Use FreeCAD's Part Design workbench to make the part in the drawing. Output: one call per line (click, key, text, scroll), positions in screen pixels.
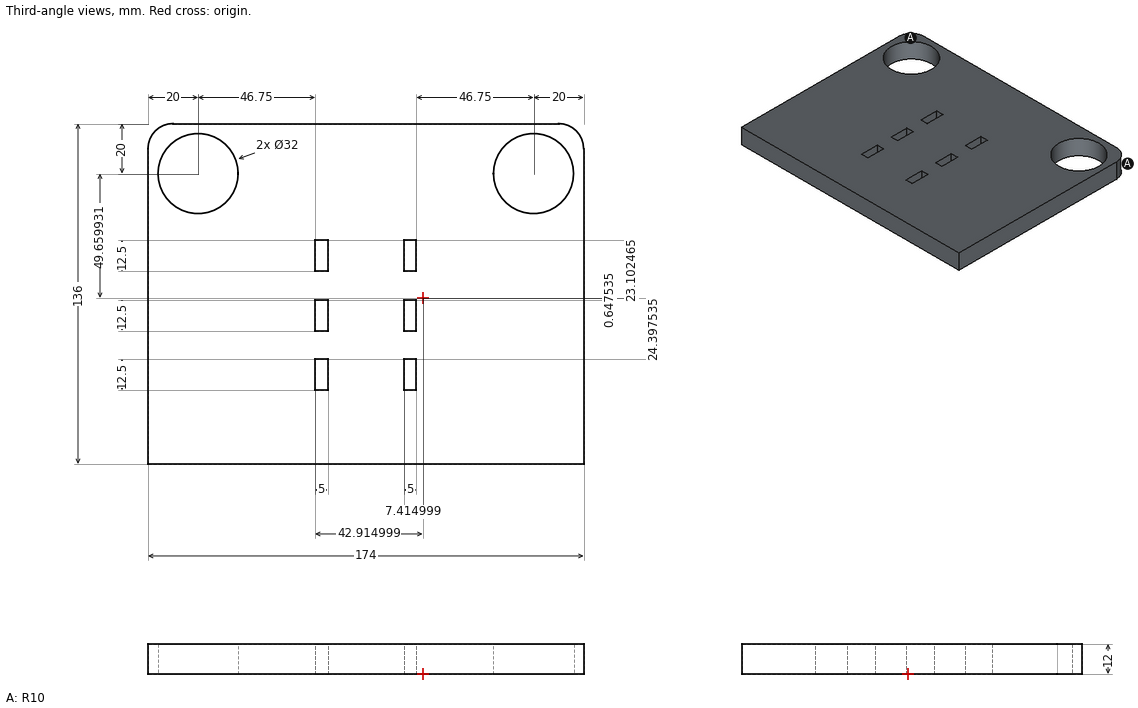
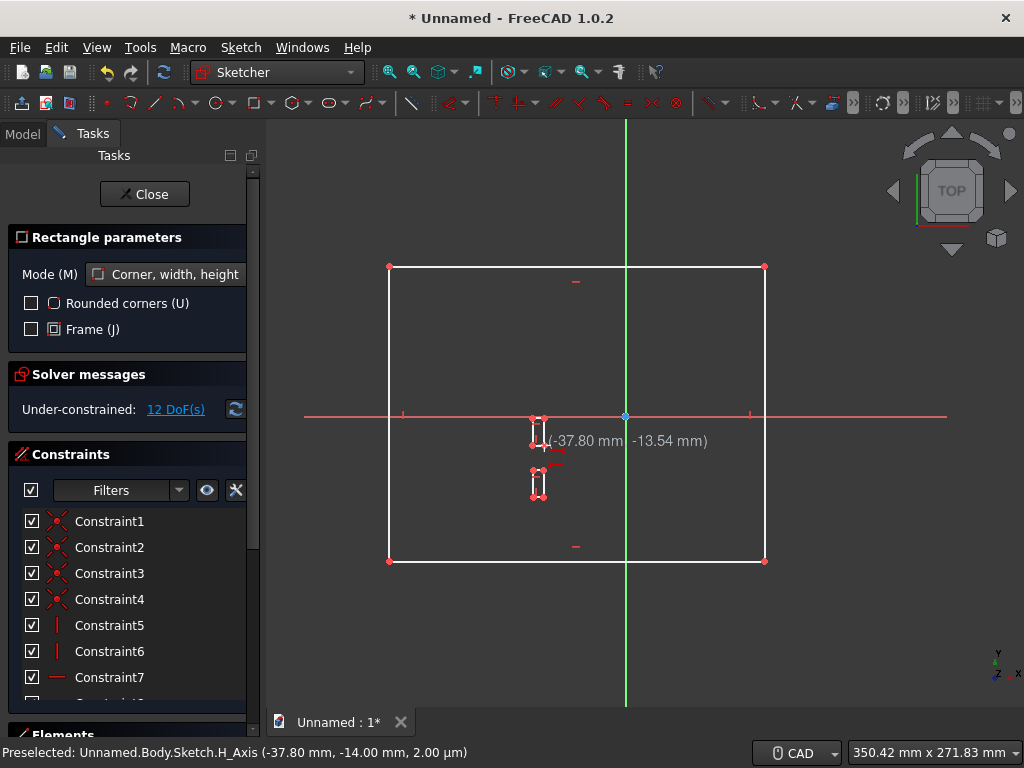
scroll(610, 469, up, 2)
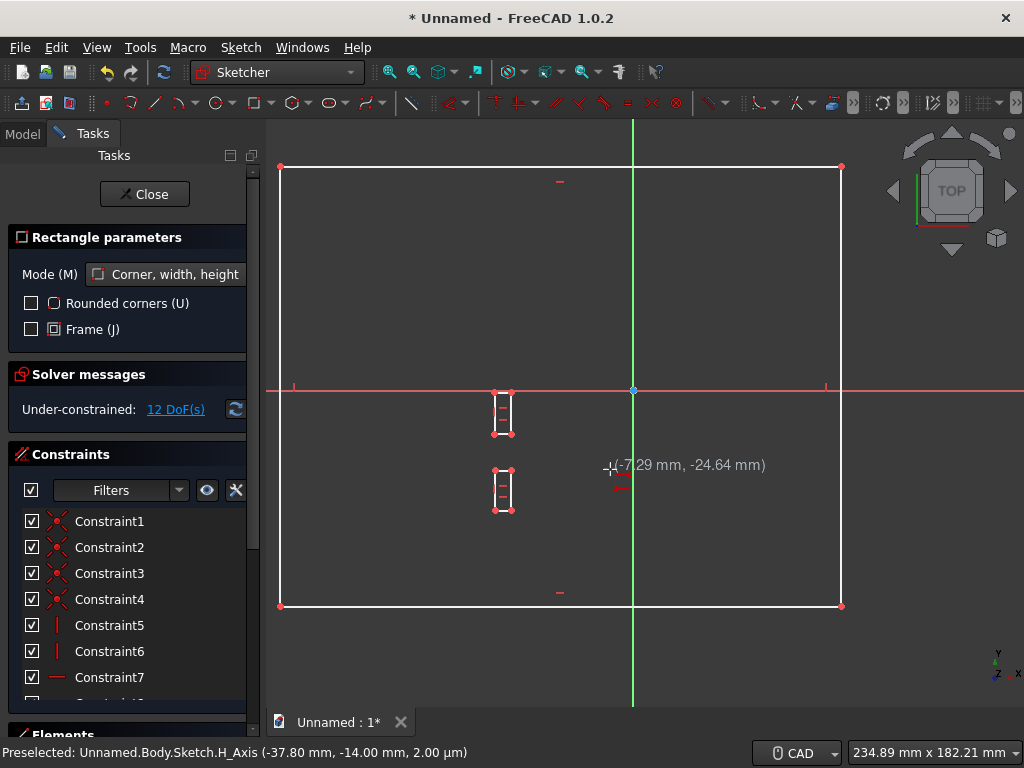
click(609, 469)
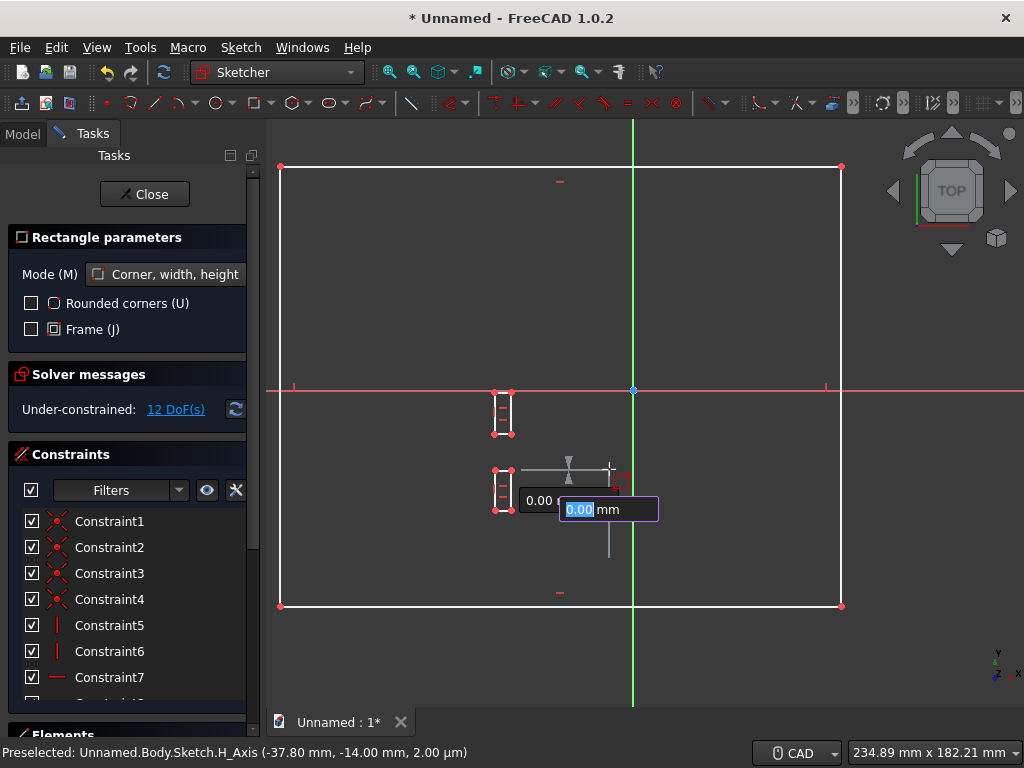
scroll(625, 510, up, 4)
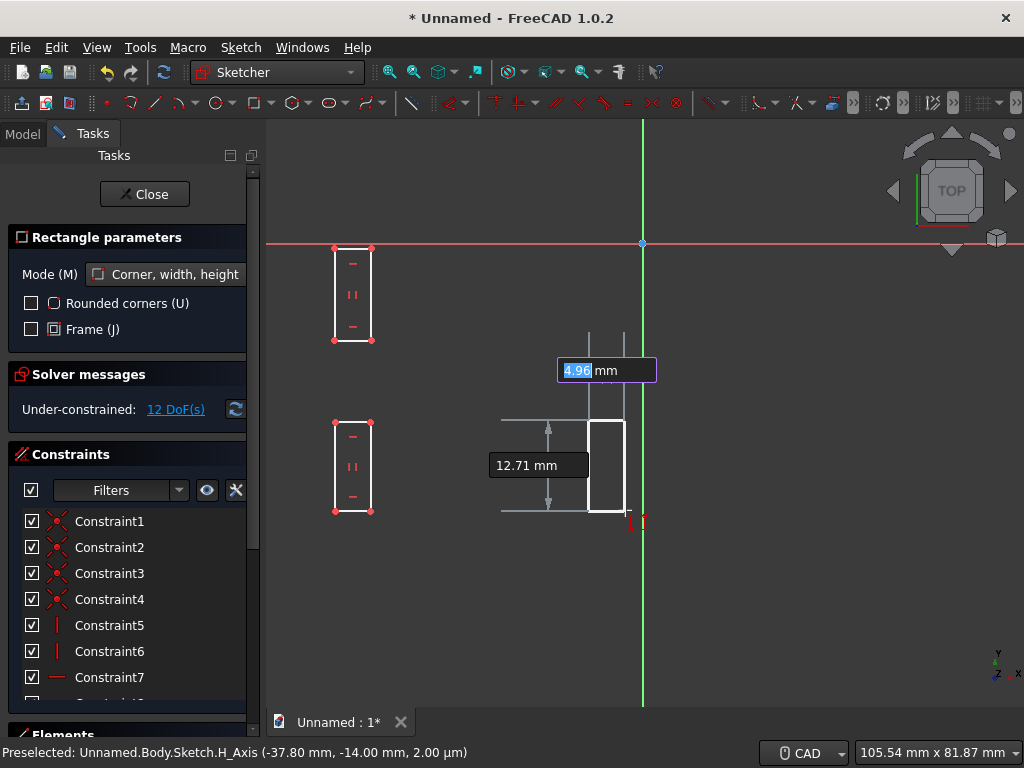
click(626, 509)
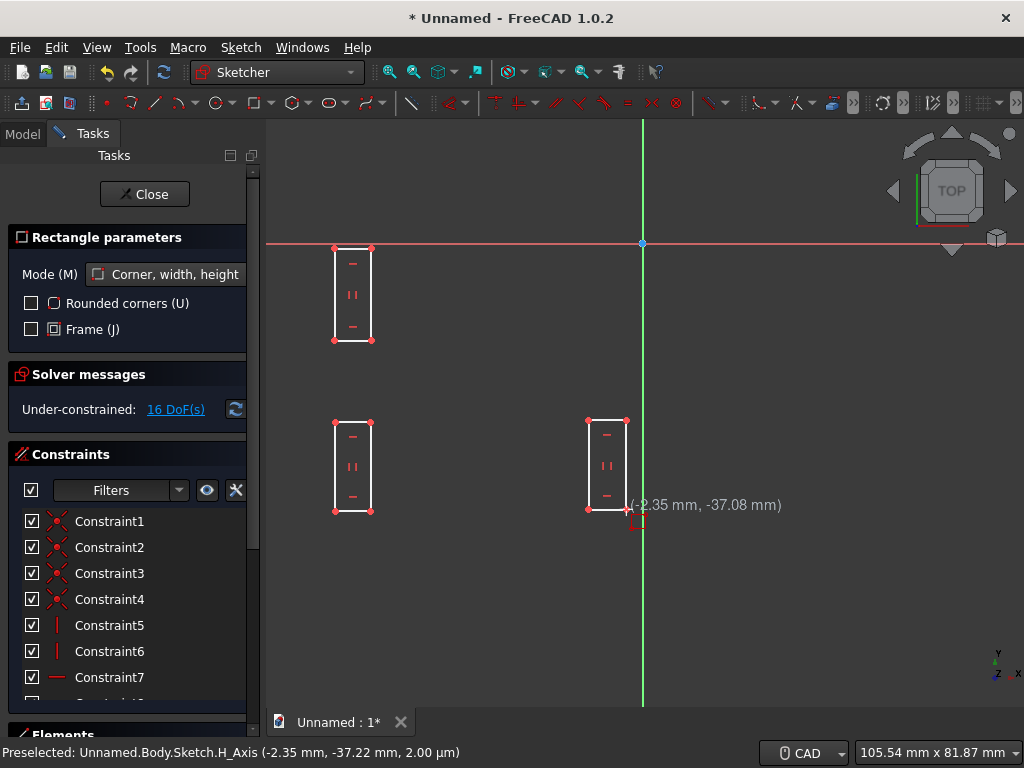
scroll(590, 248, up, 7)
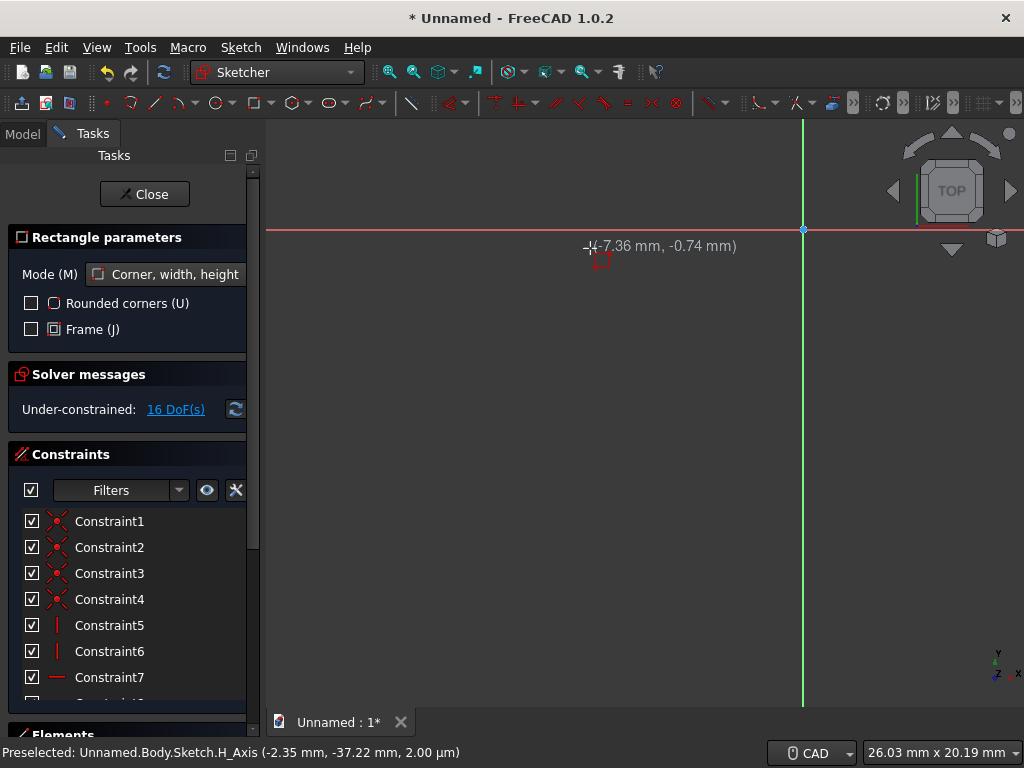
click(587, 249)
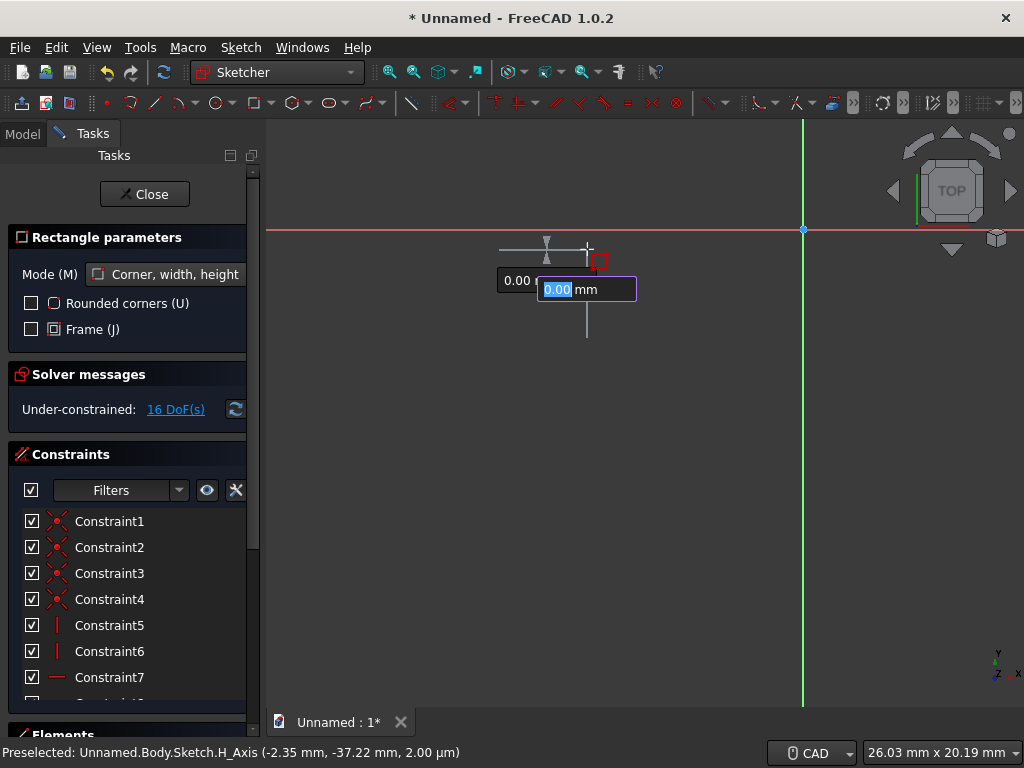
scroll(611, 432, down, 13)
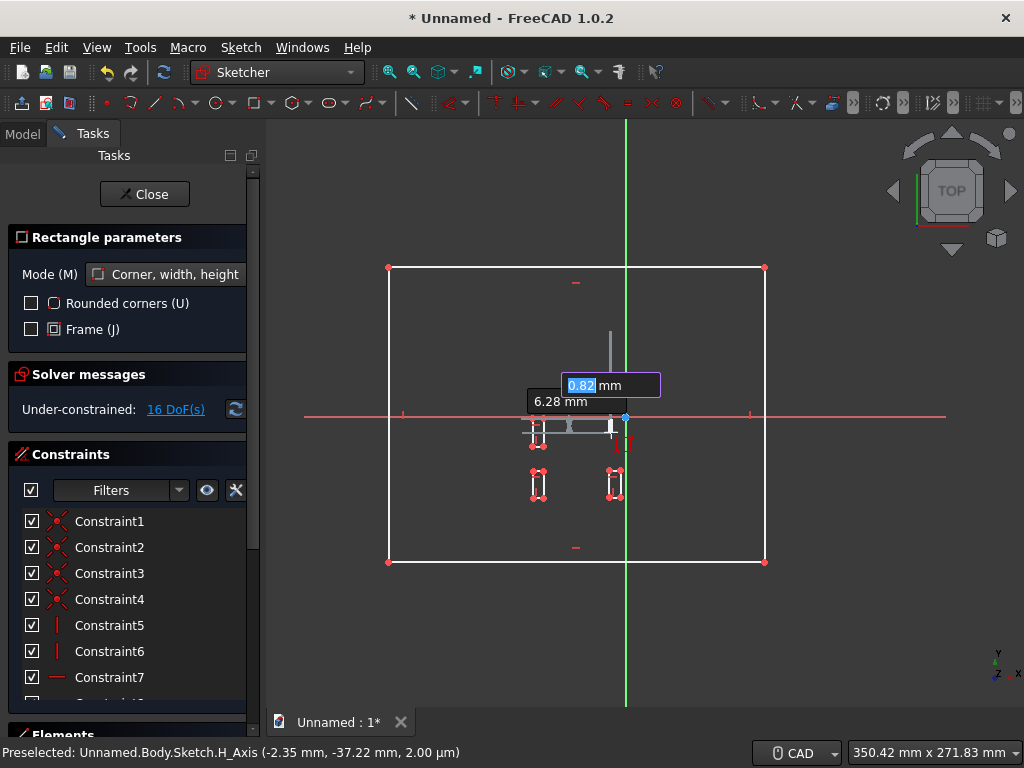
scroll(620, 446, up, 6)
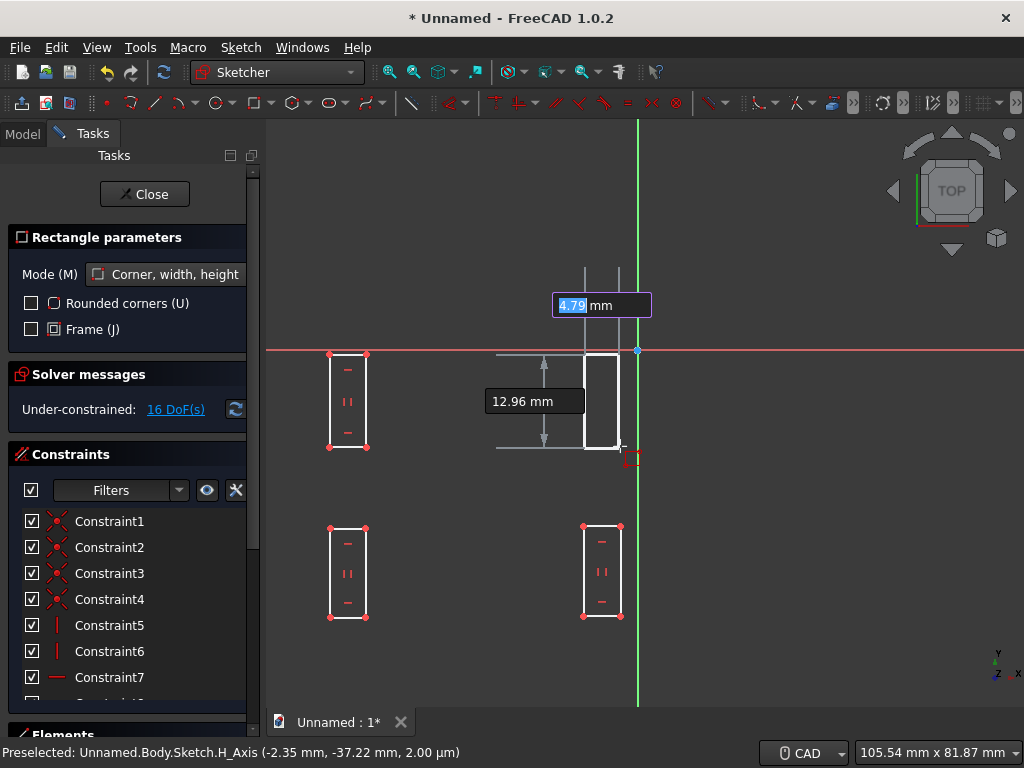
click(620, 444)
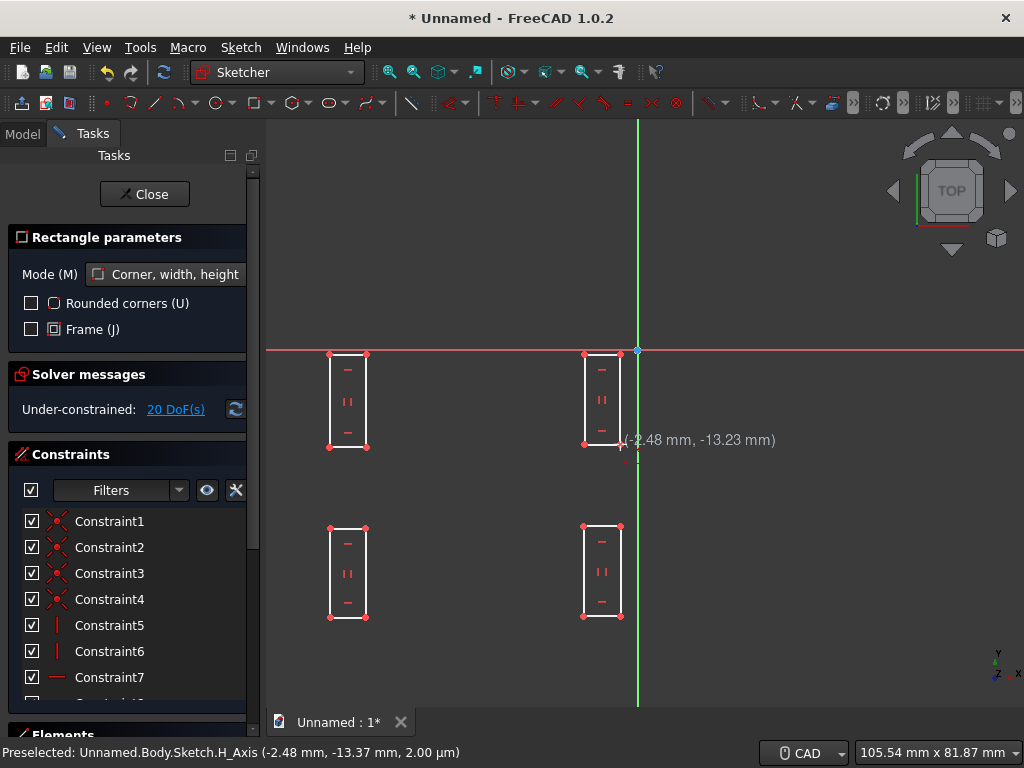
click(330, 184)
click(365, 274)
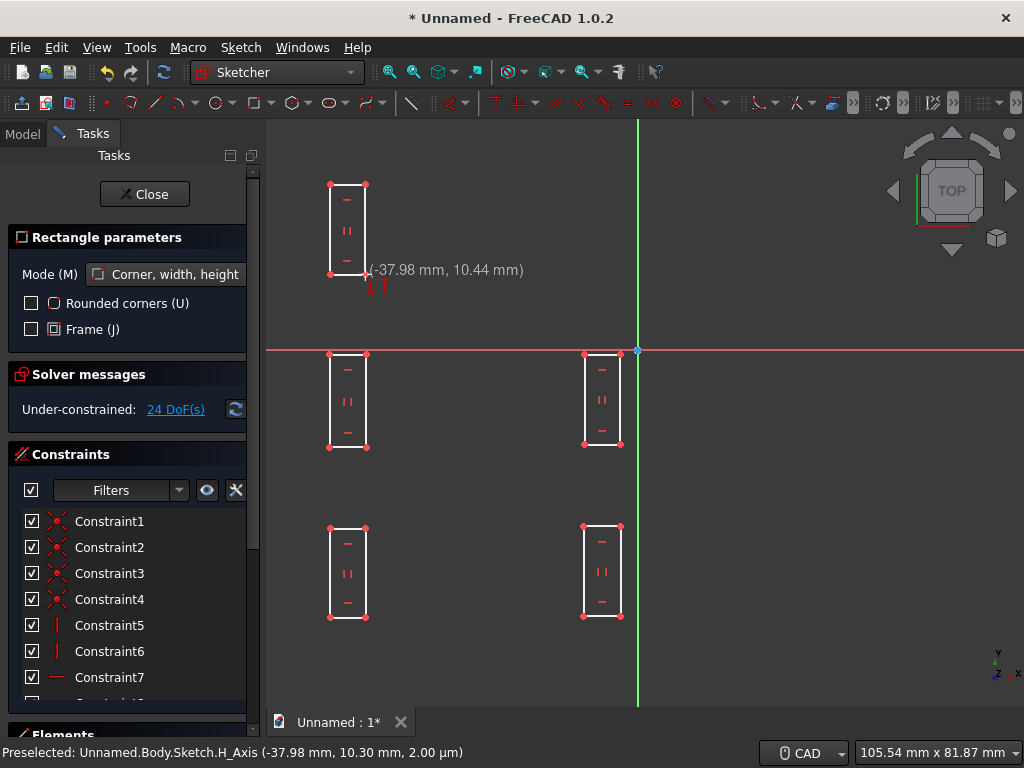
click(585, 184)
click(620, 274)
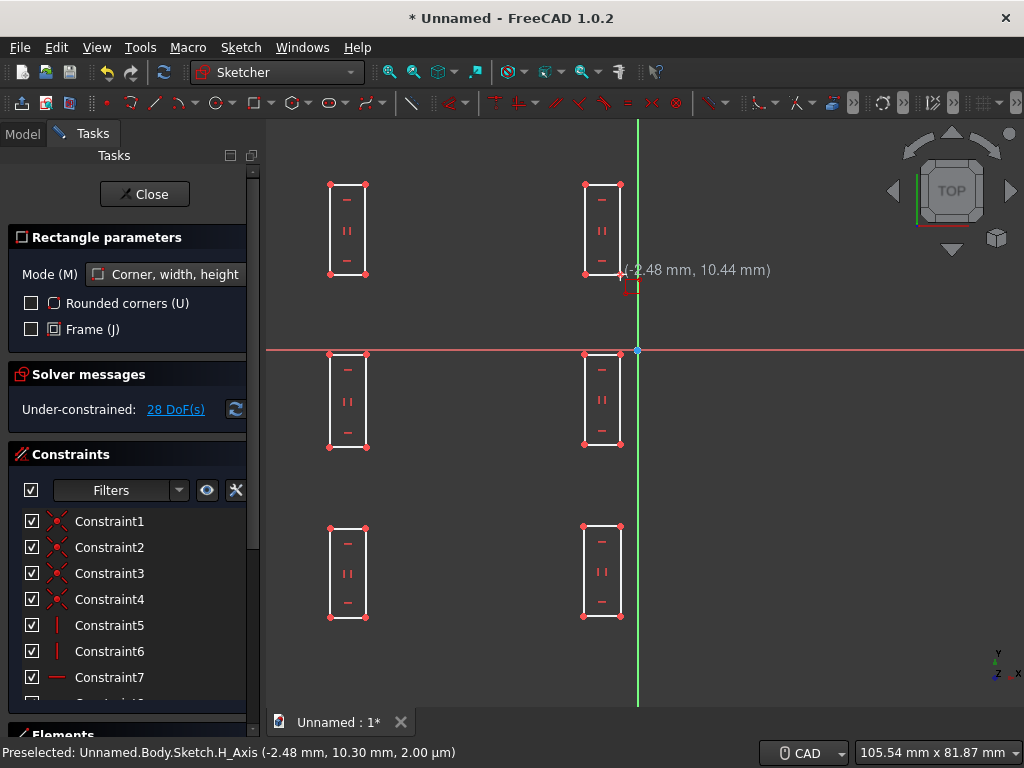
click(216, 104)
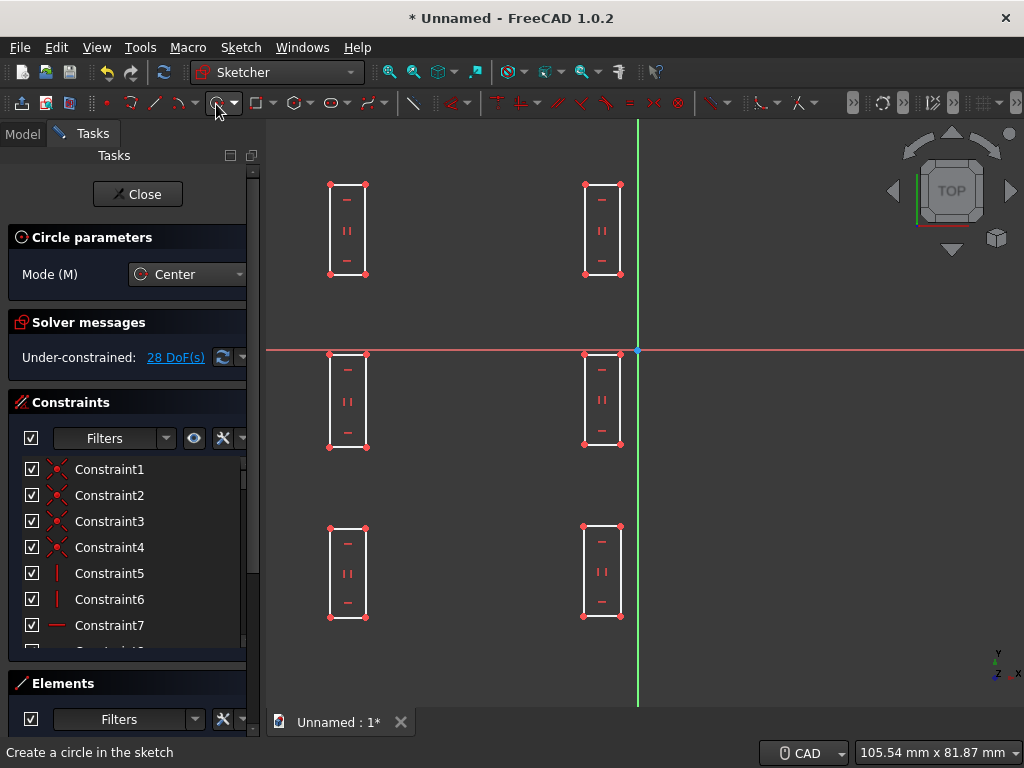
scroll(620, 445, down, 6)